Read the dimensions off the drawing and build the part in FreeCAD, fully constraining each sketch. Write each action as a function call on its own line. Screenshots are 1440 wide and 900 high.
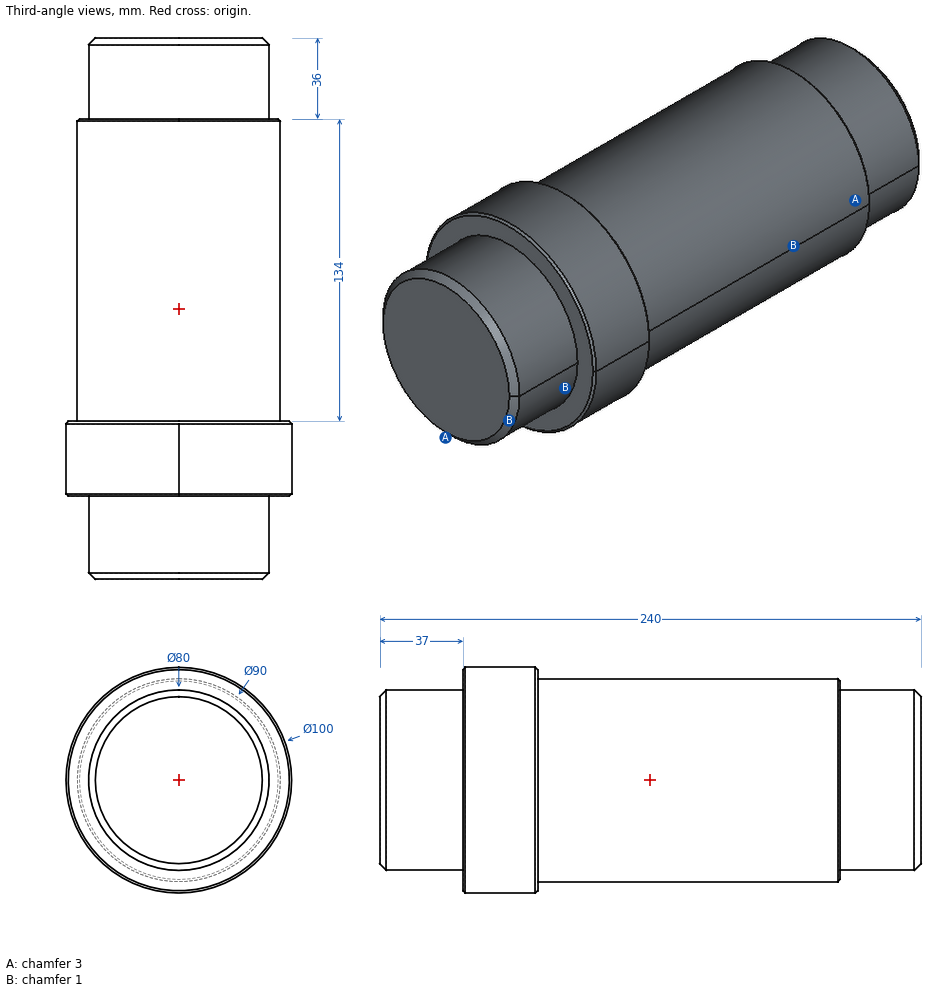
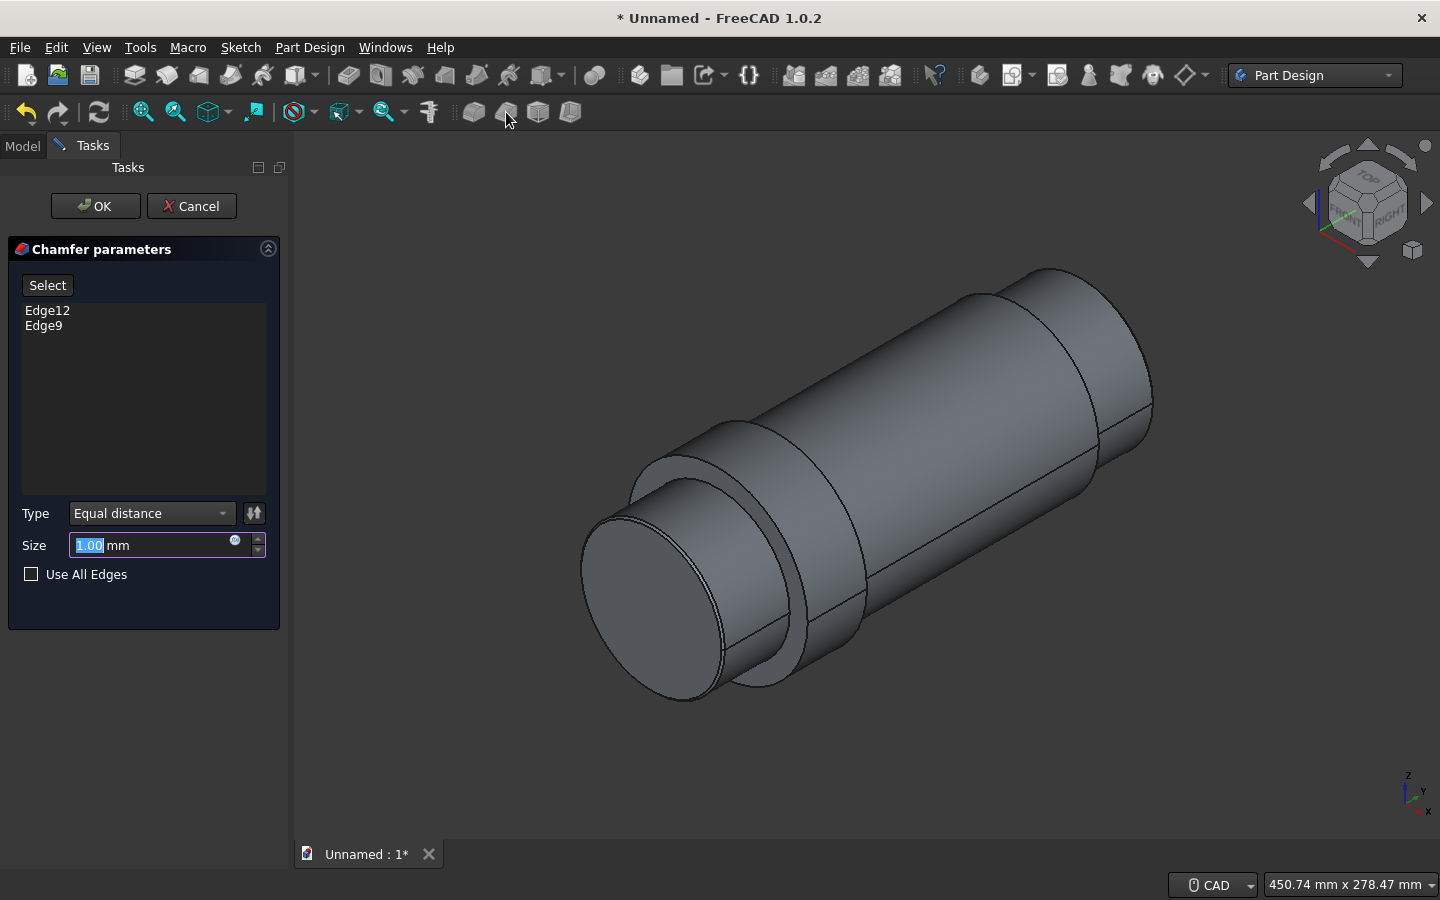
text(3)
key(Tab)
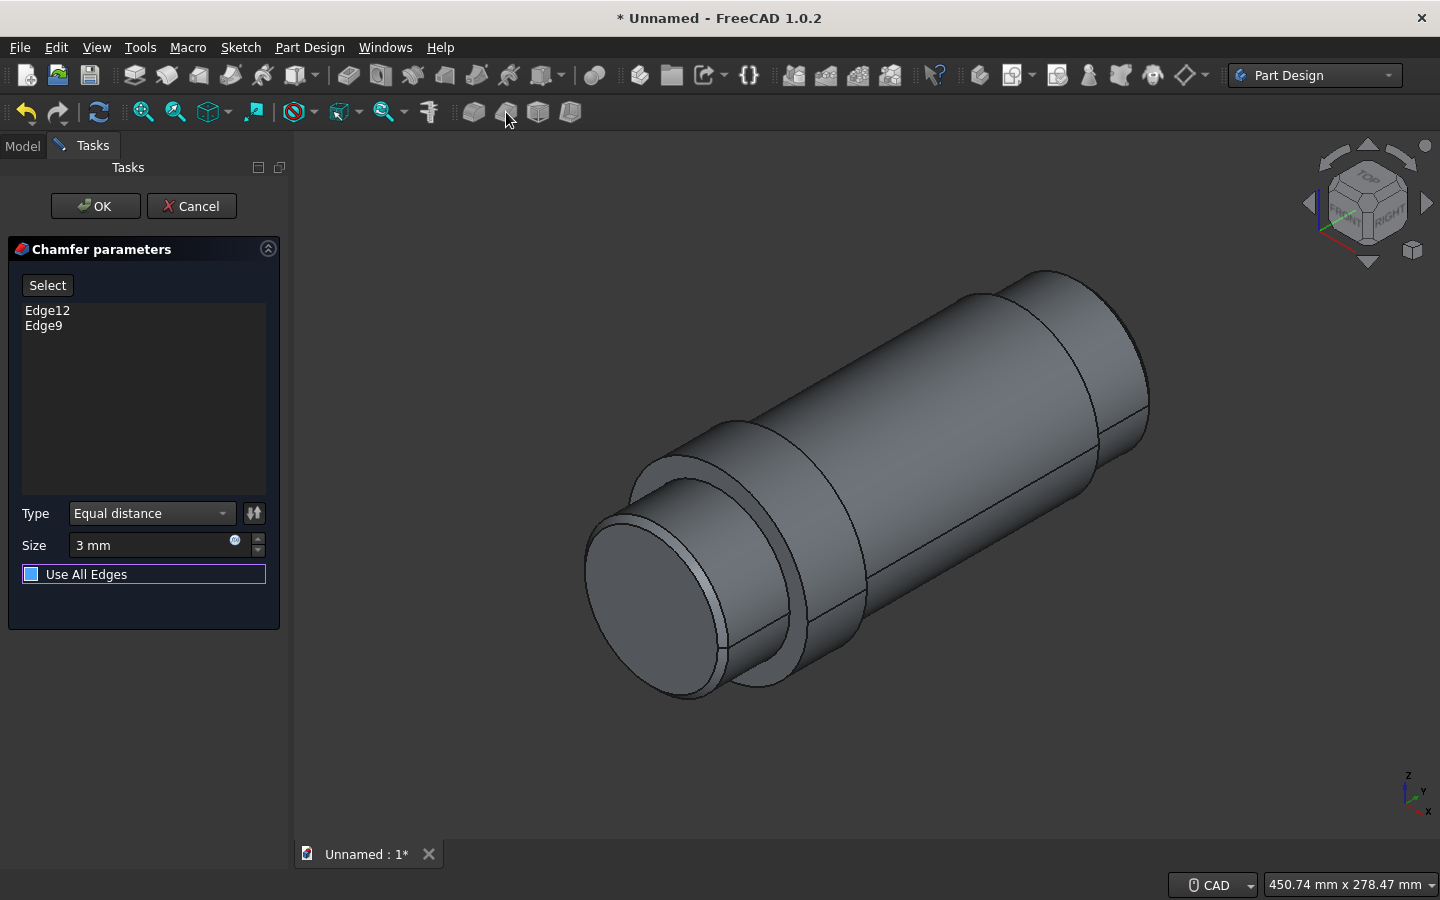
click(96, 206)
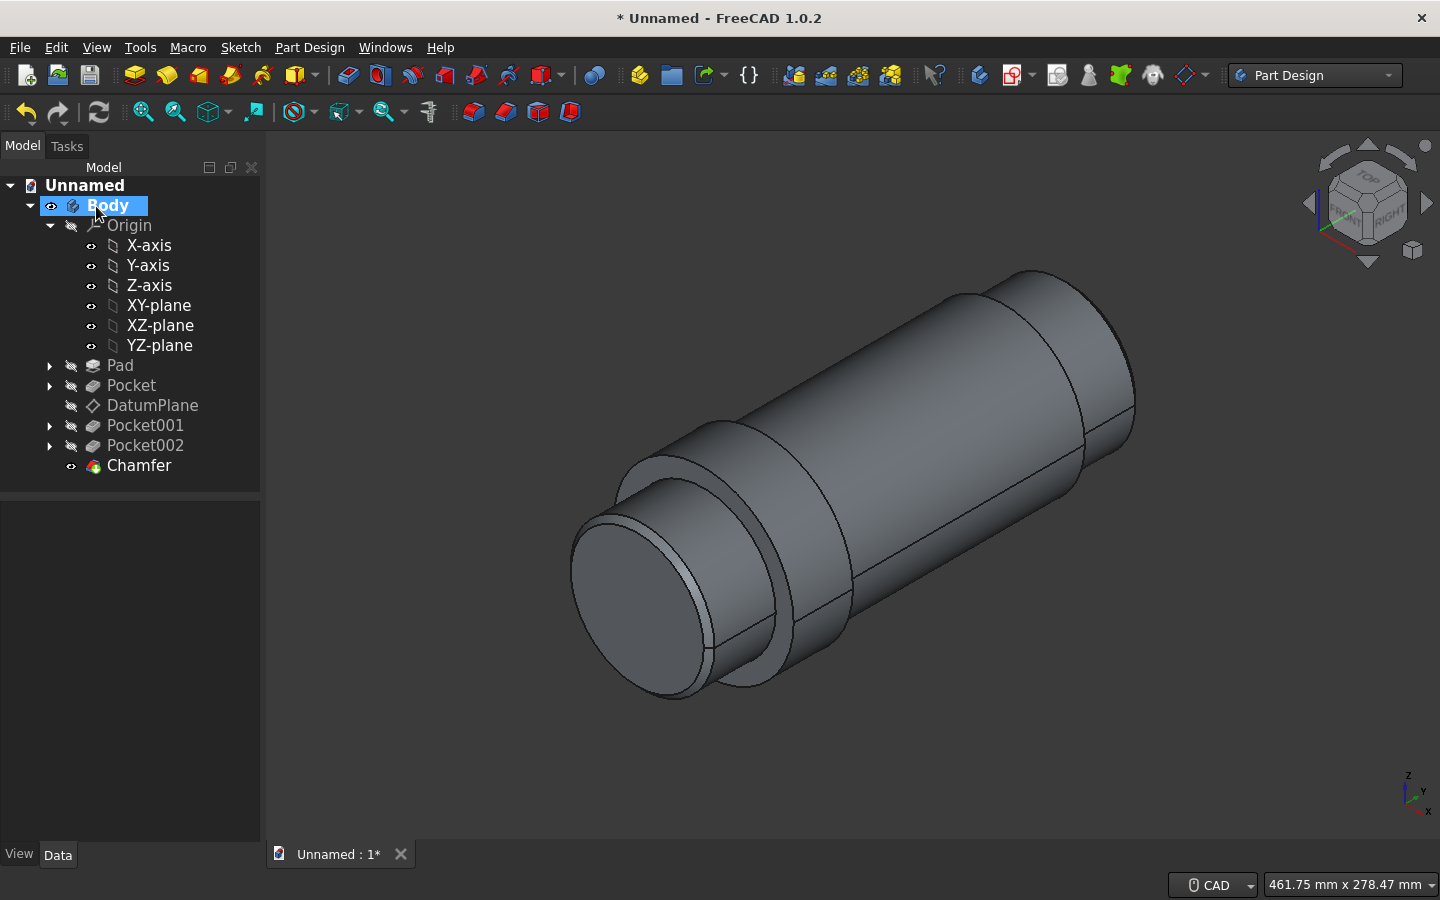
click(676, 455)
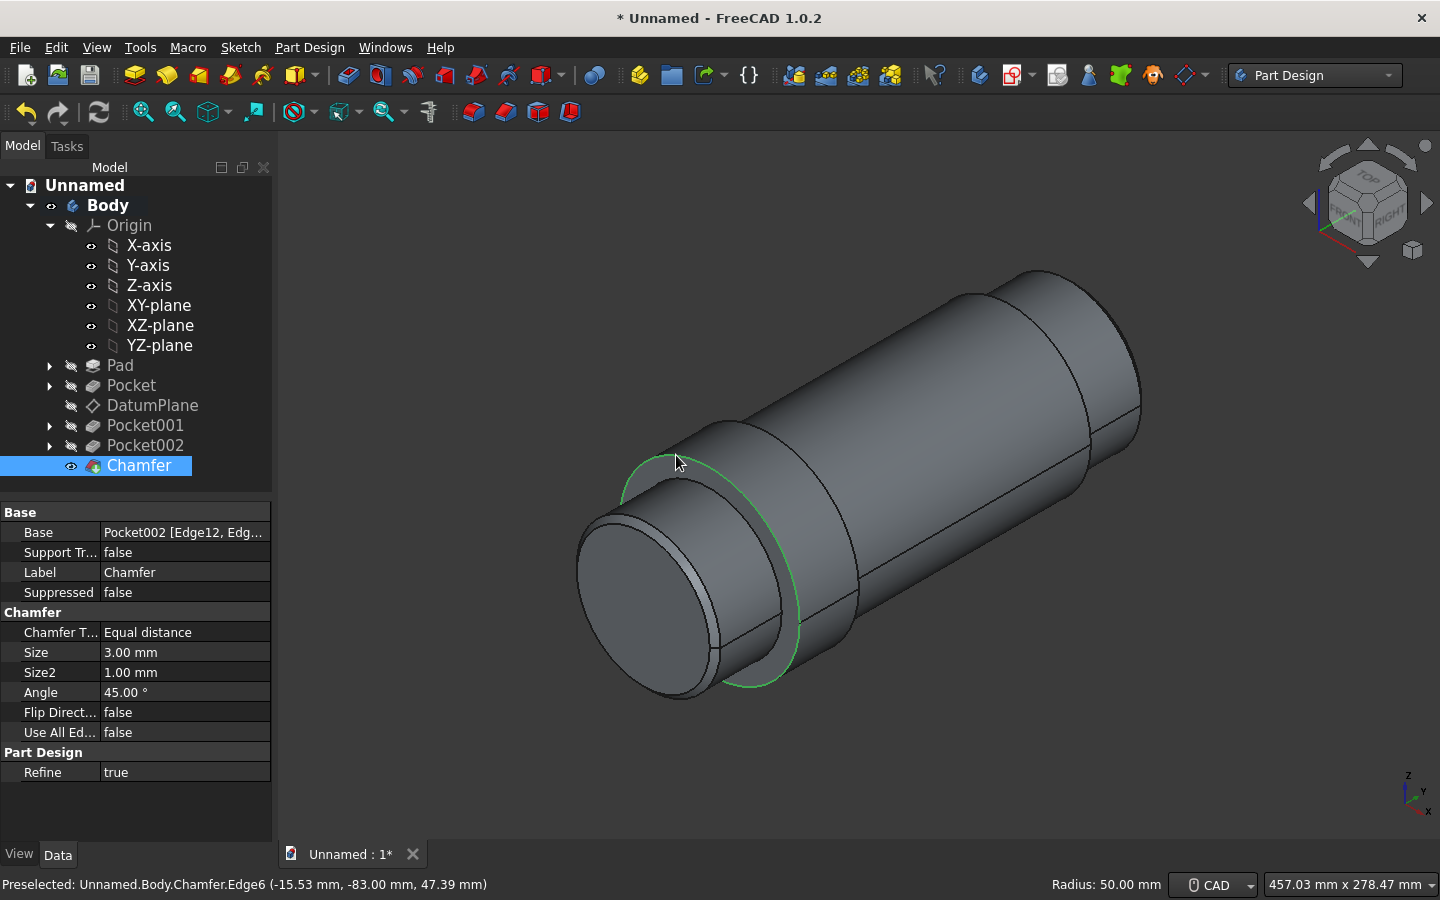
key(2)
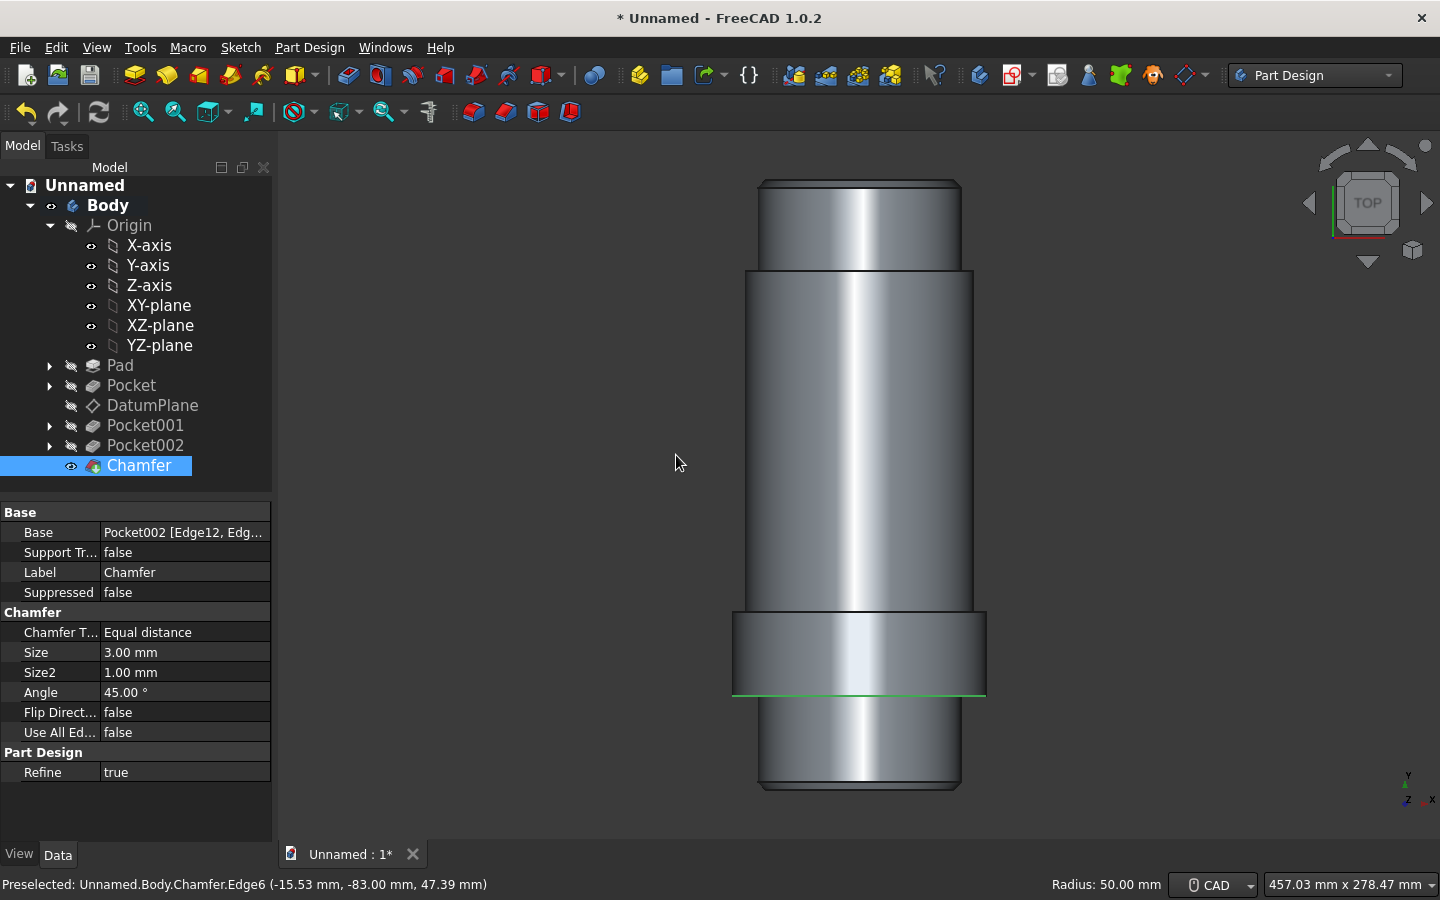
click(756, 611, ctrl)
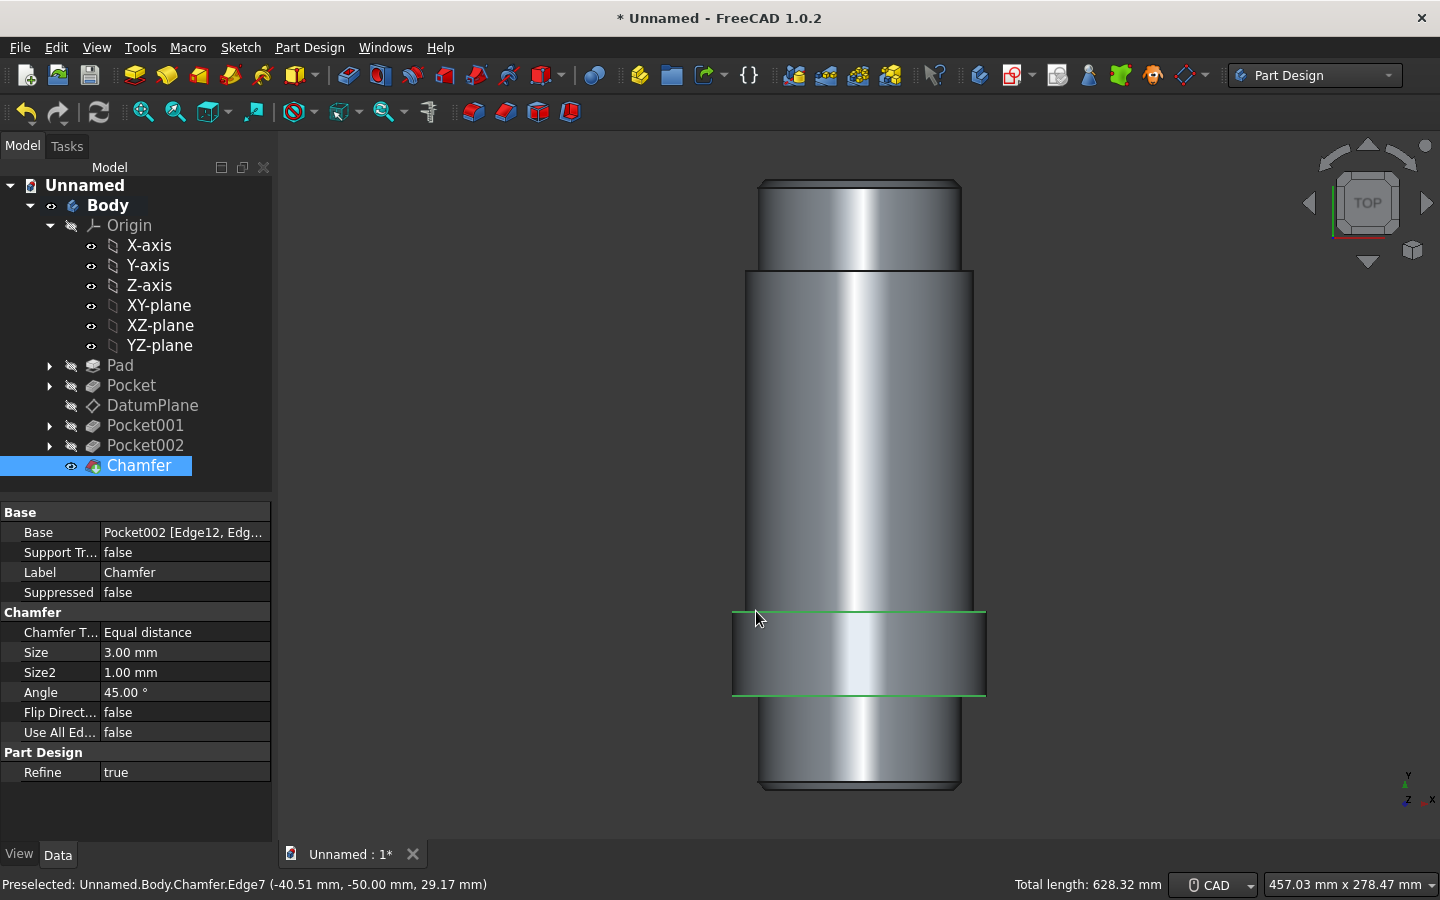
click(766, 270, ctrl)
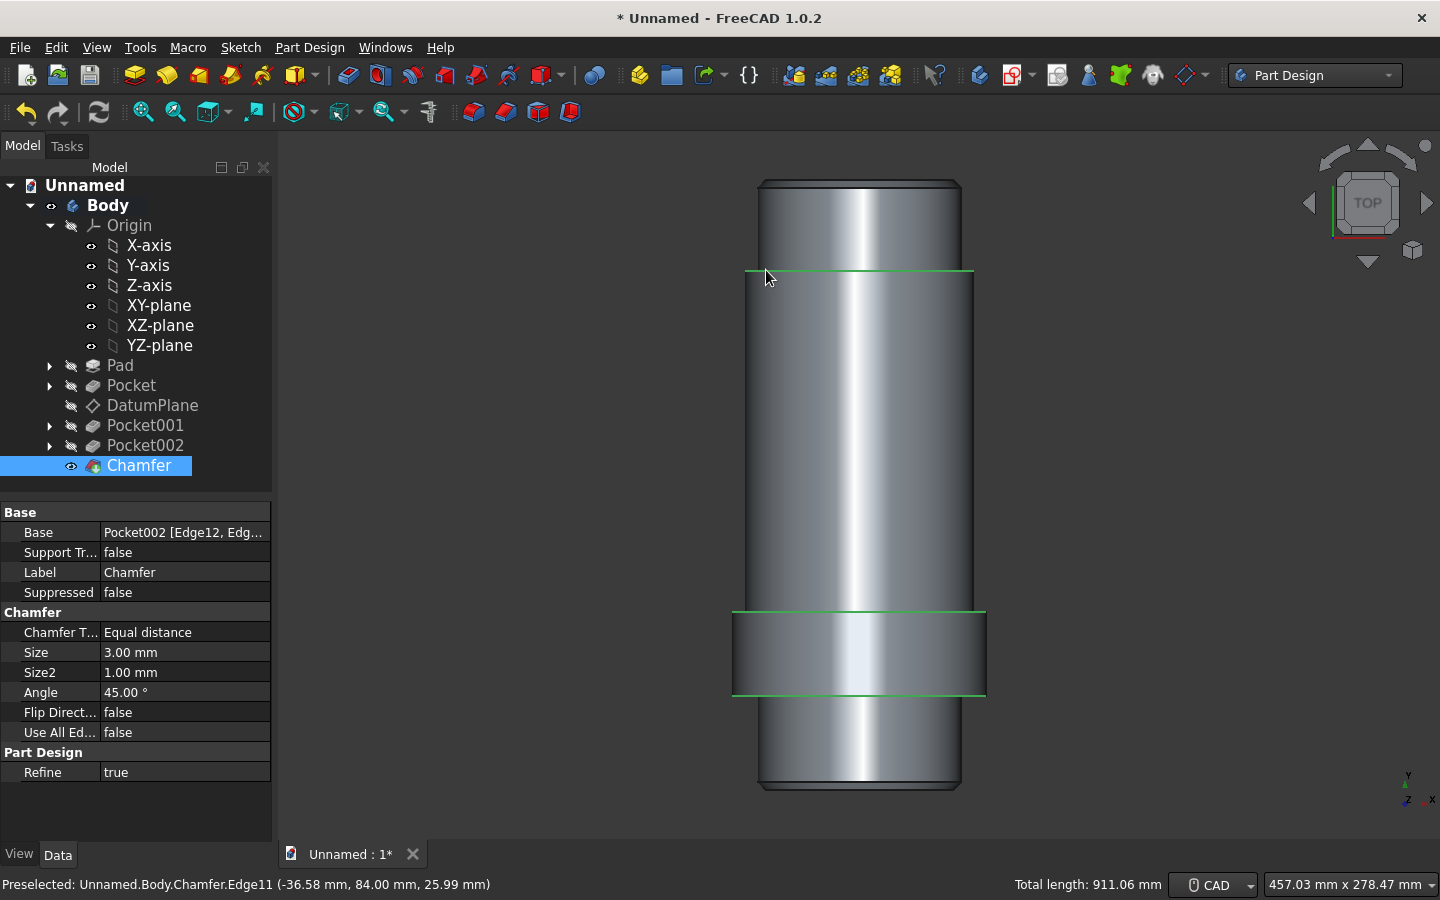
click(506, 112)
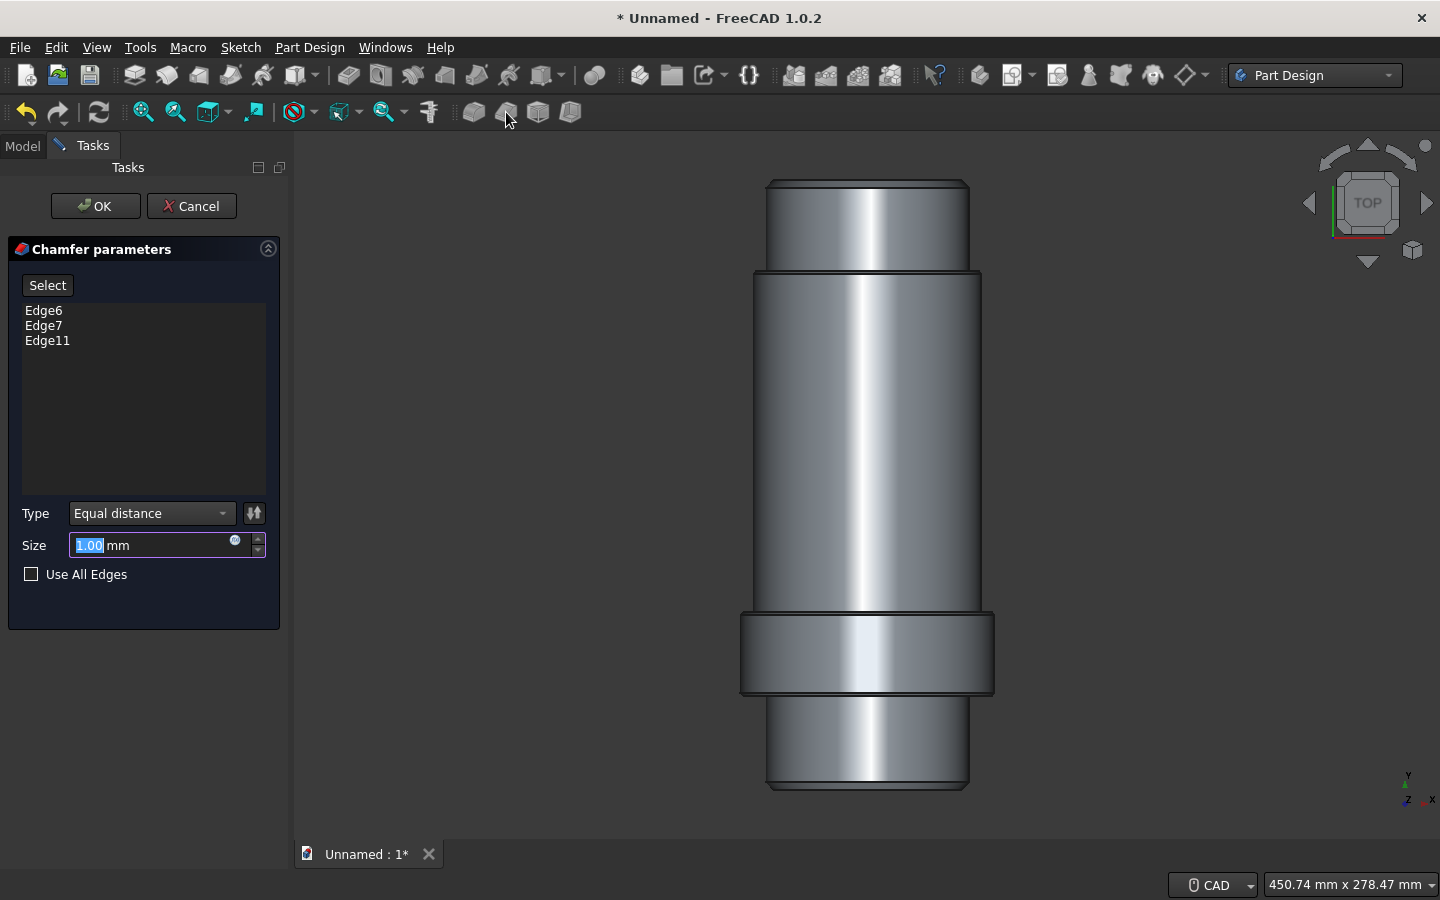
text(1)
key(Tab)